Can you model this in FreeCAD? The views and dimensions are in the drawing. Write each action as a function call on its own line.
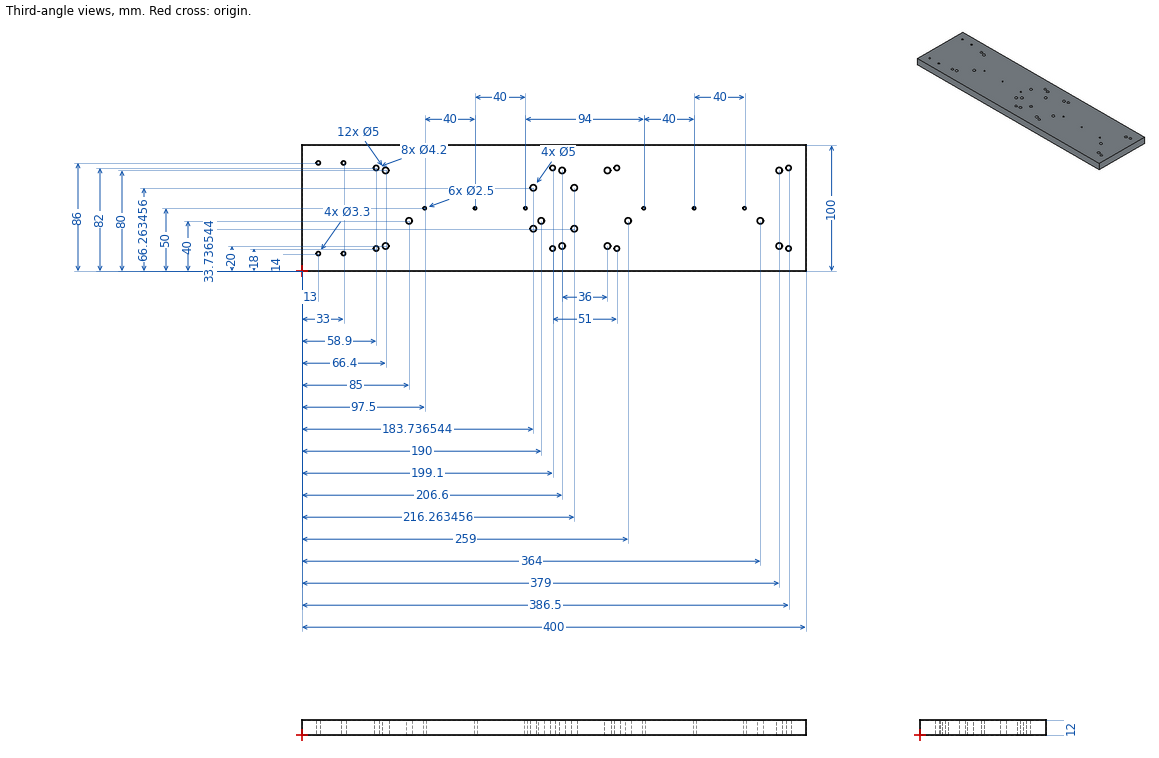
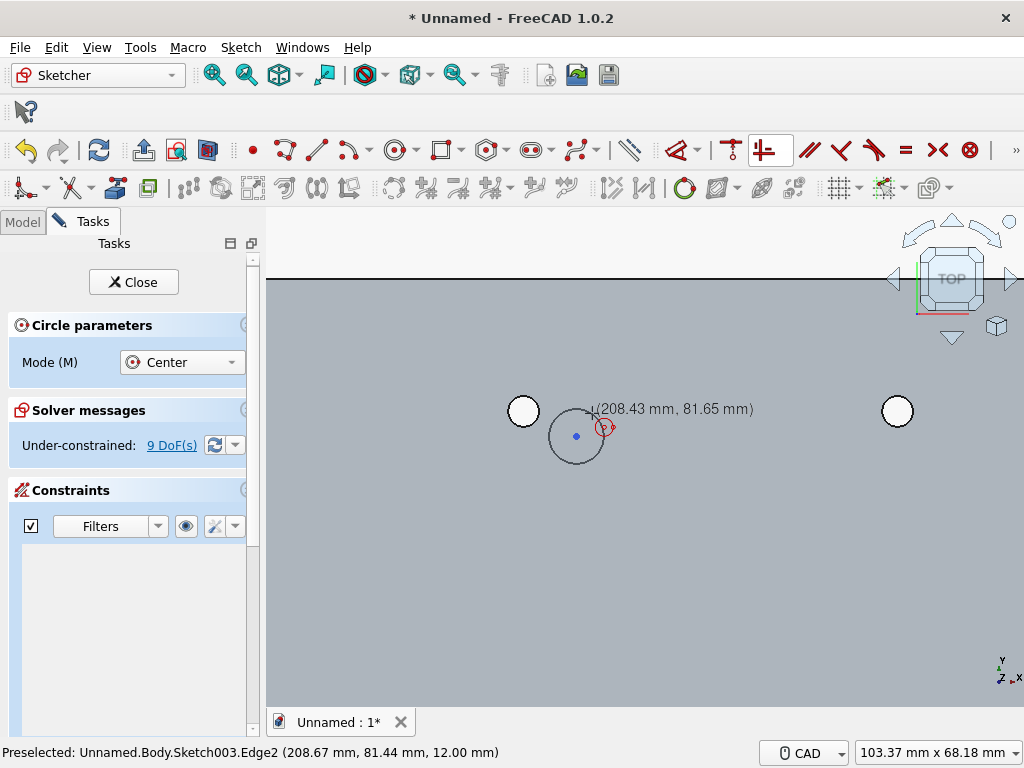
scroll(594, 417, down, 10)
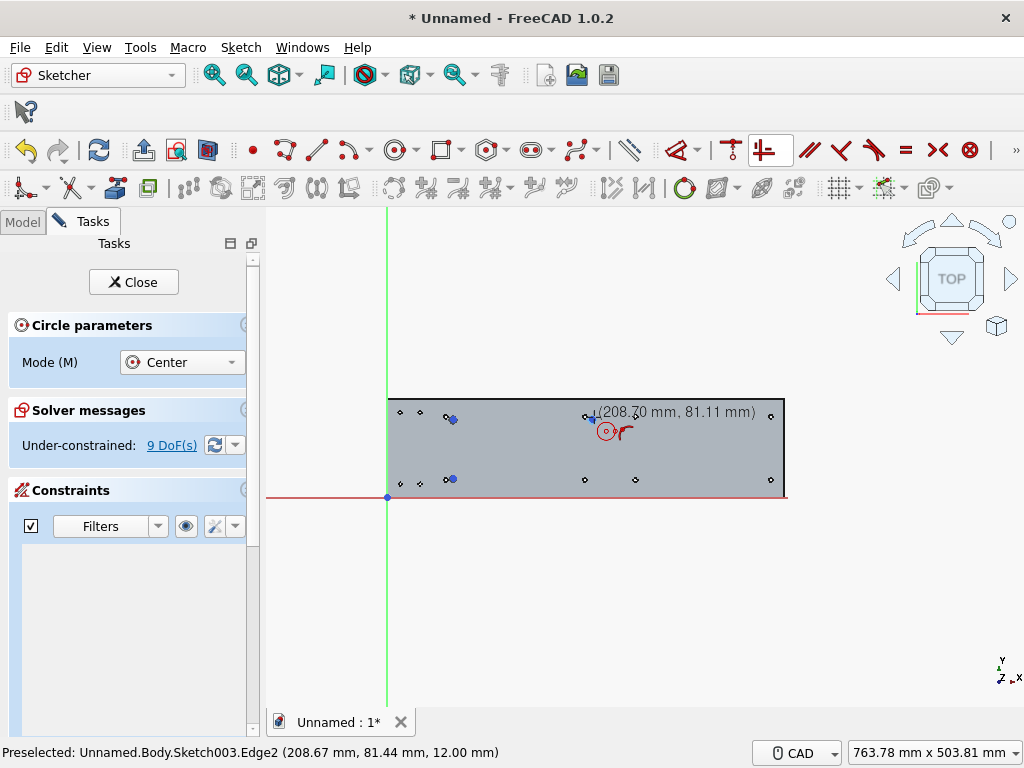
scroll(592, 478, up, 12)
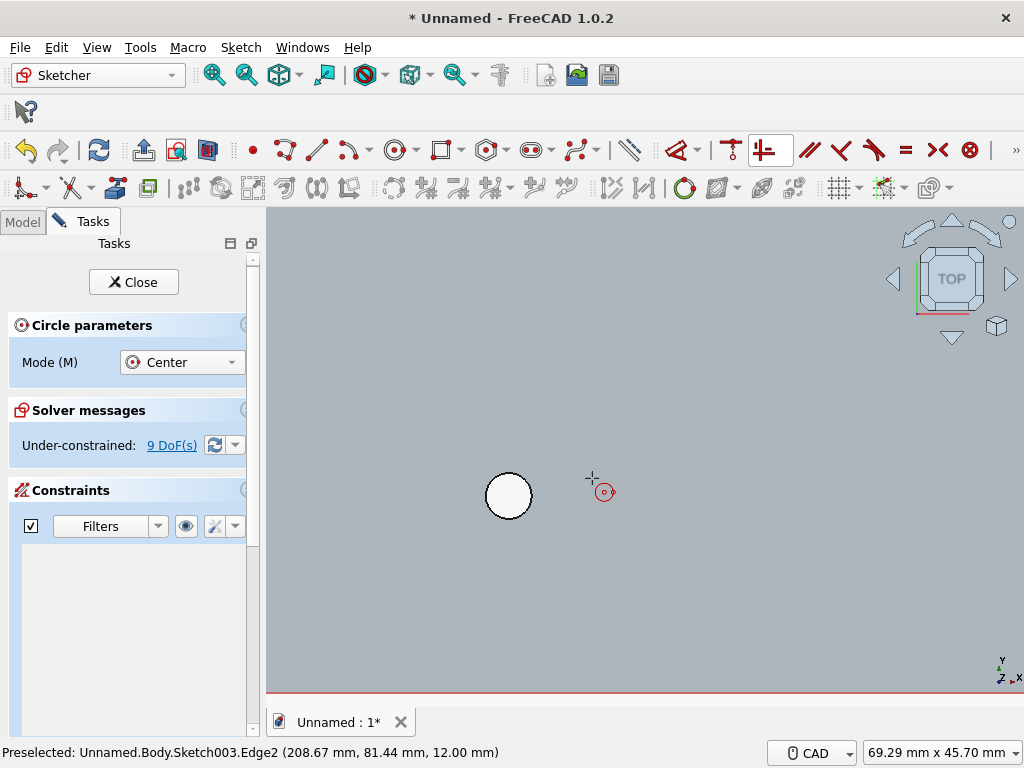
scroll(592, 478, down, 12)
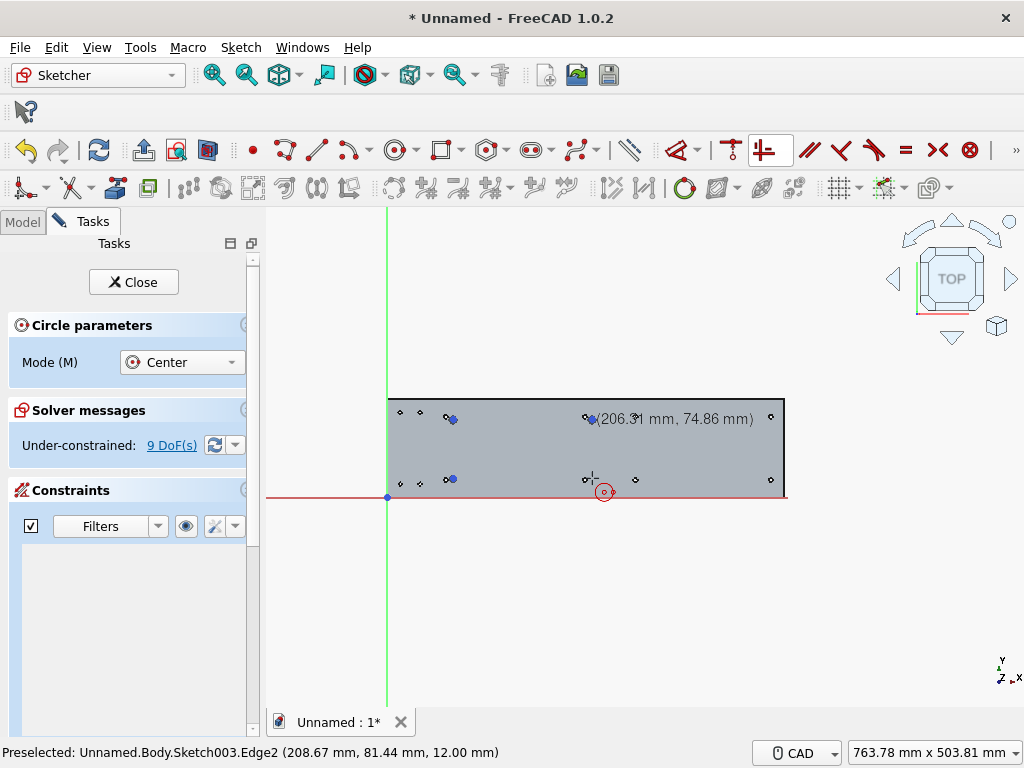
click(592, 478)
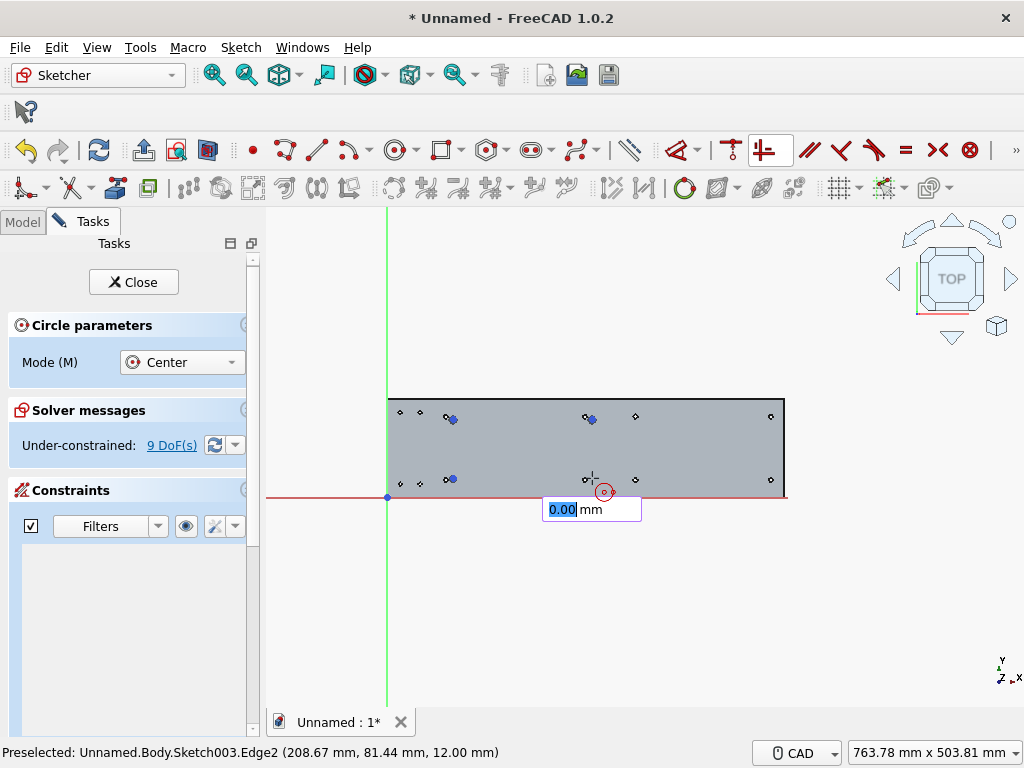
scroll(594, 476, up, 10)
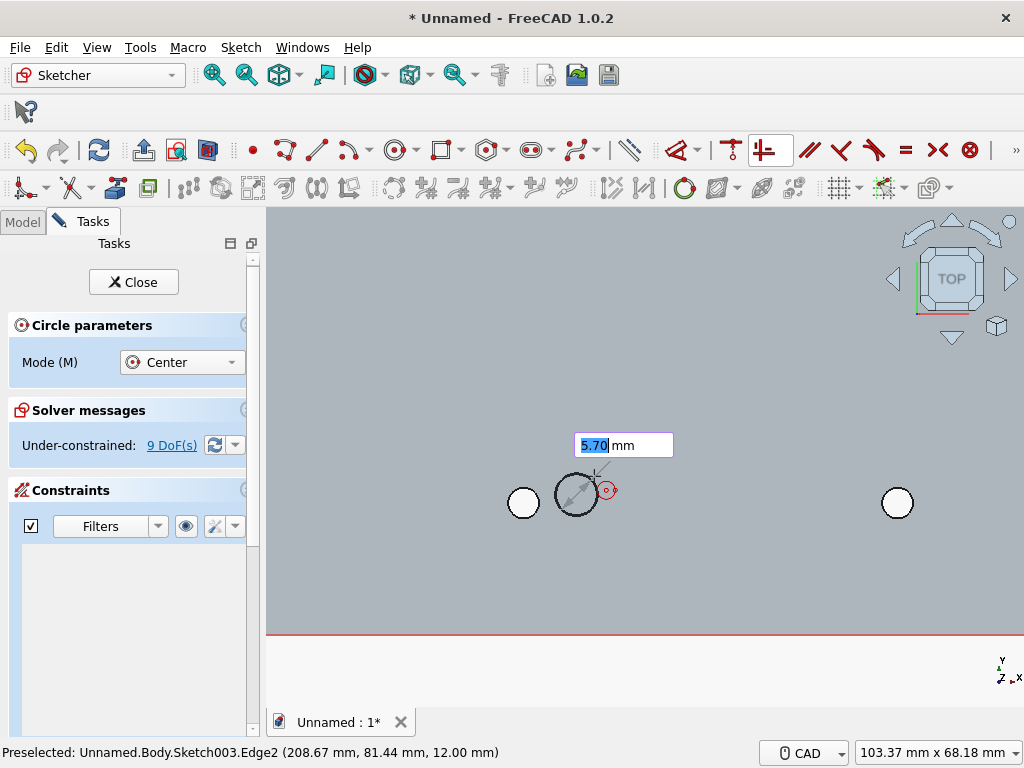
click(592, 475)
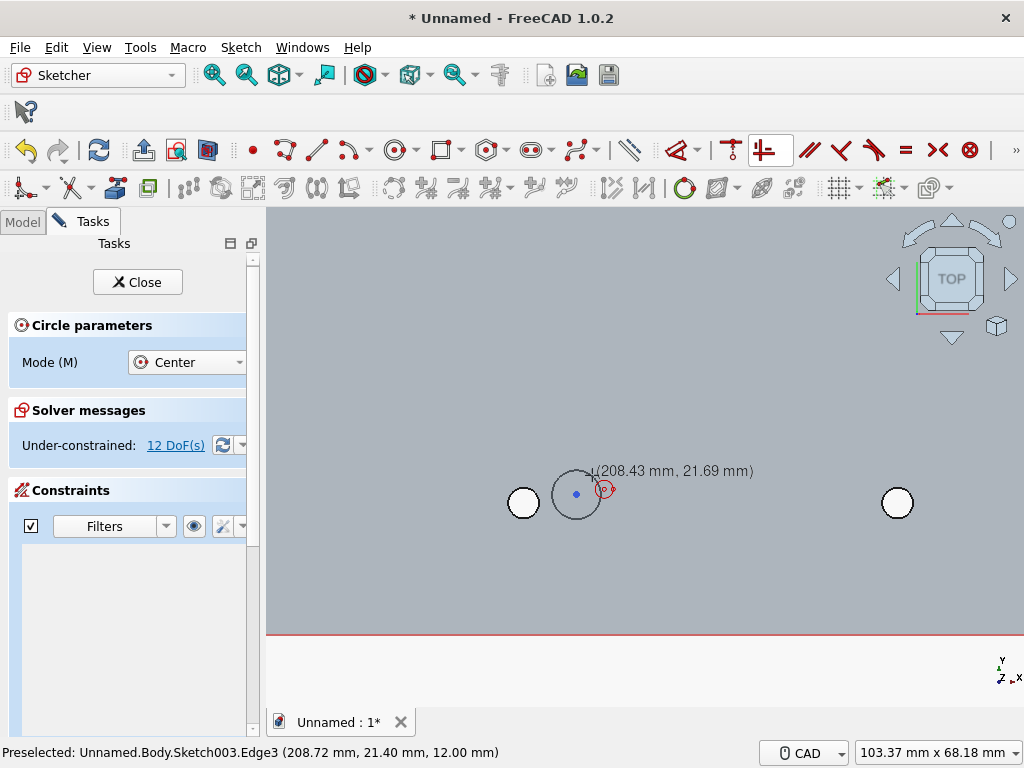
scroll(843, 488, up, 2)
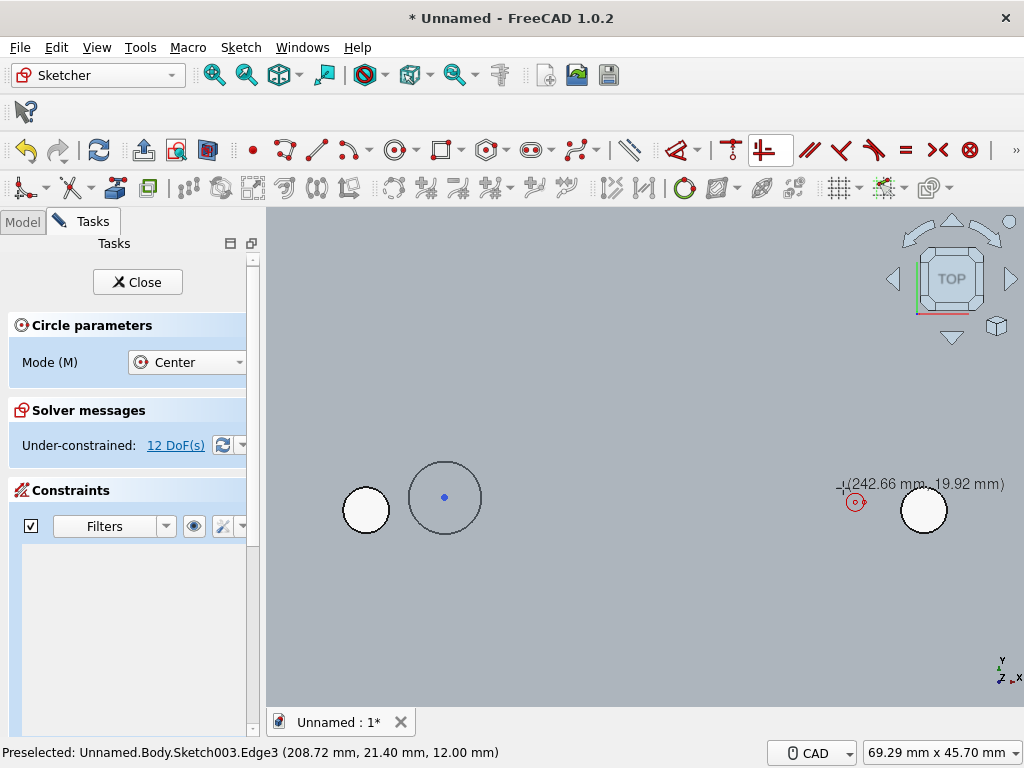
scroll(607, 477, down, 12)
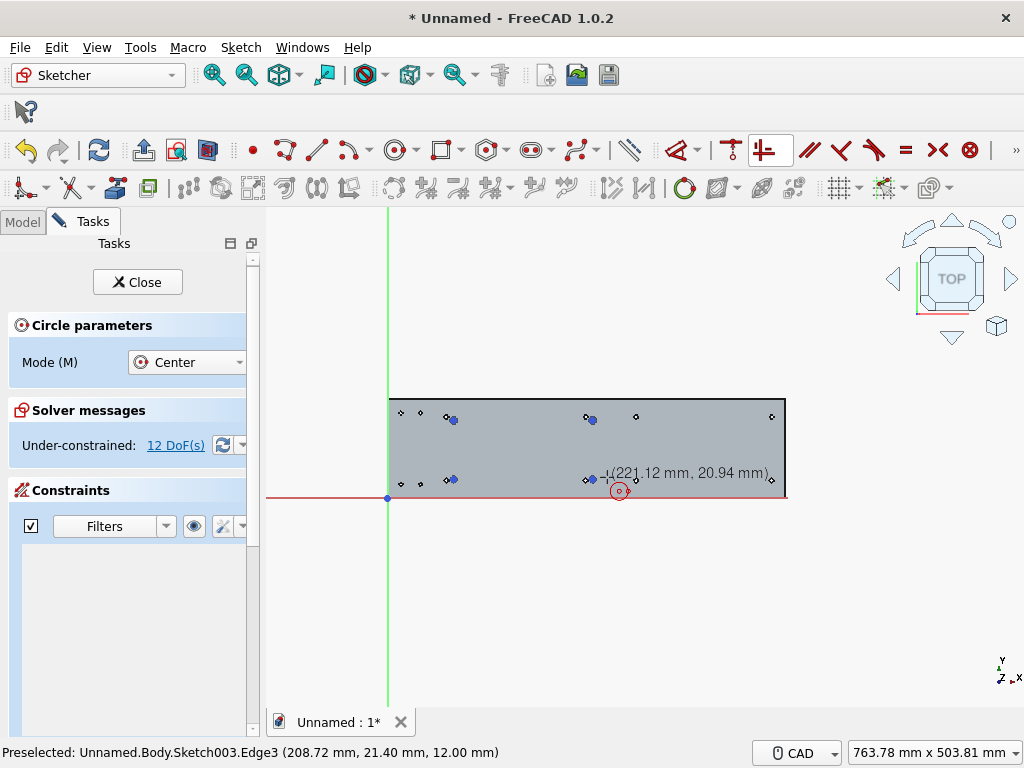
click(629, 479)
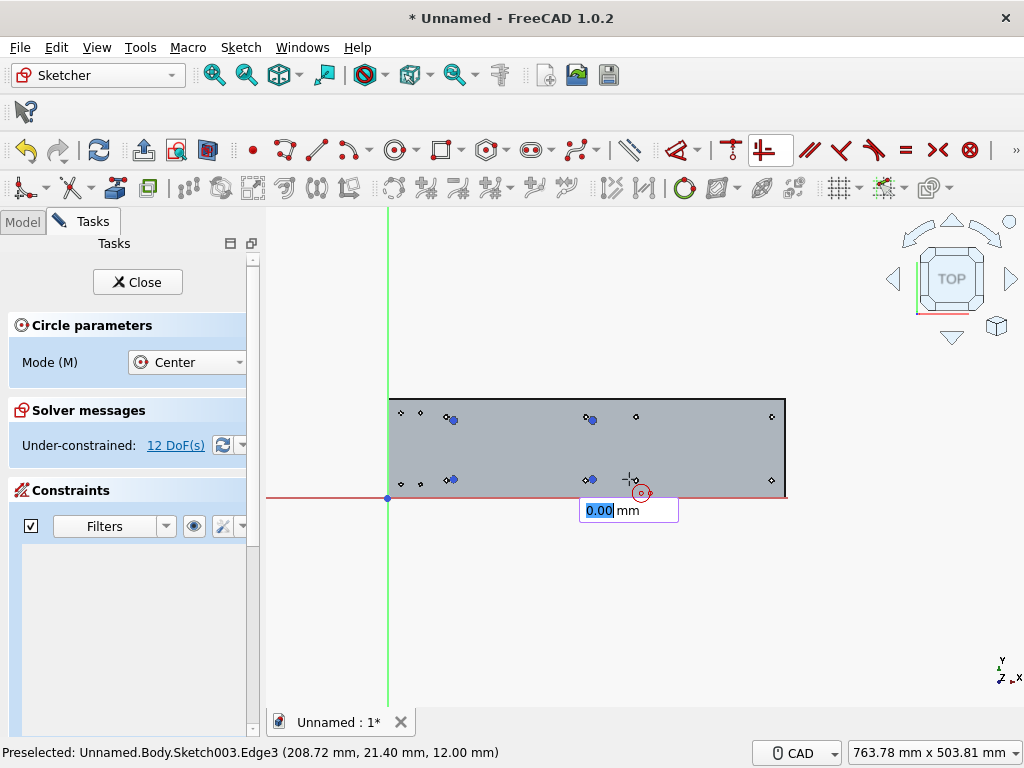
scroll(630, 477, up, 10)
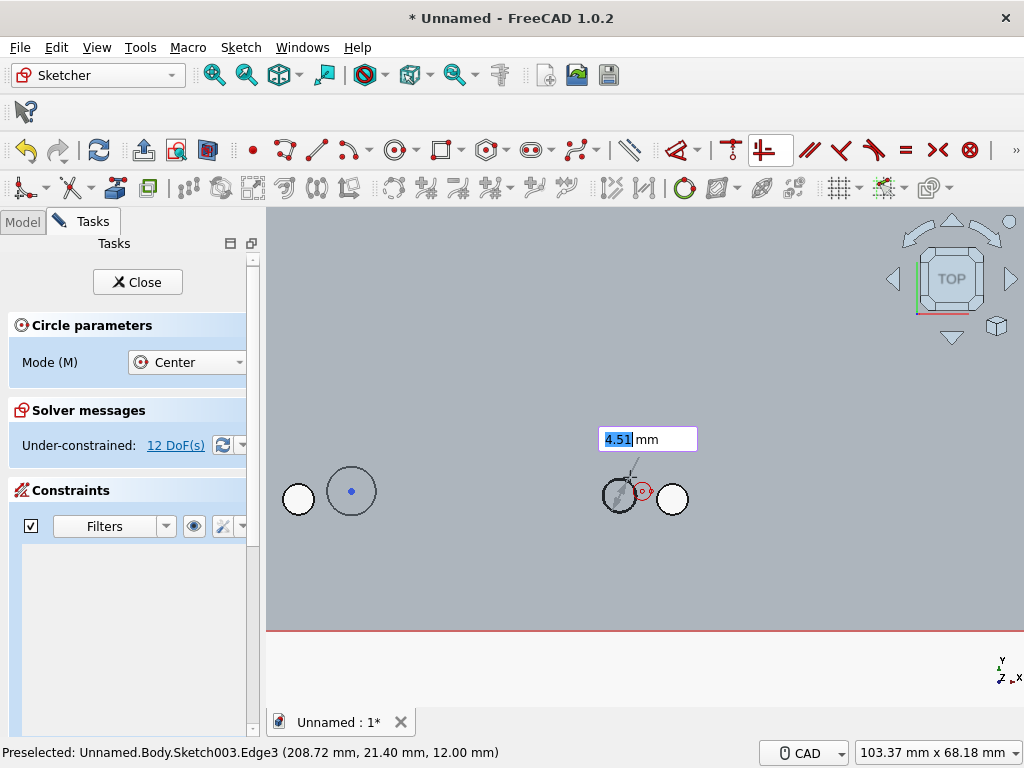
click(630, 472)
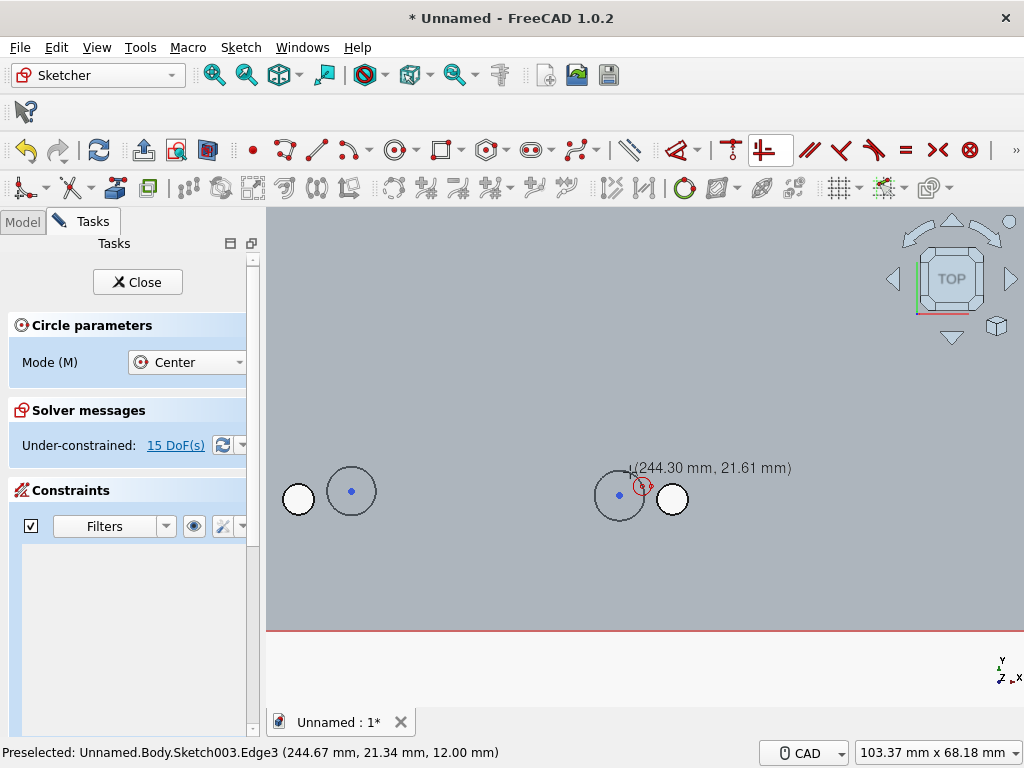
scroll(630, 477, down, 10)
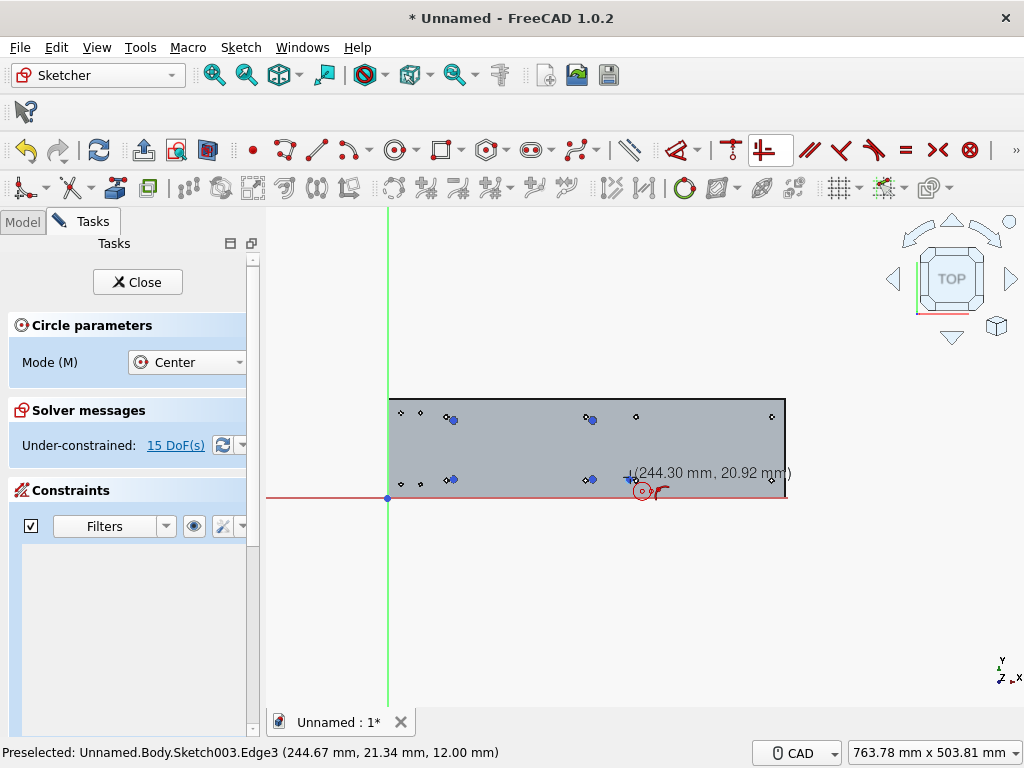
scroll(629, 419, up, 12)